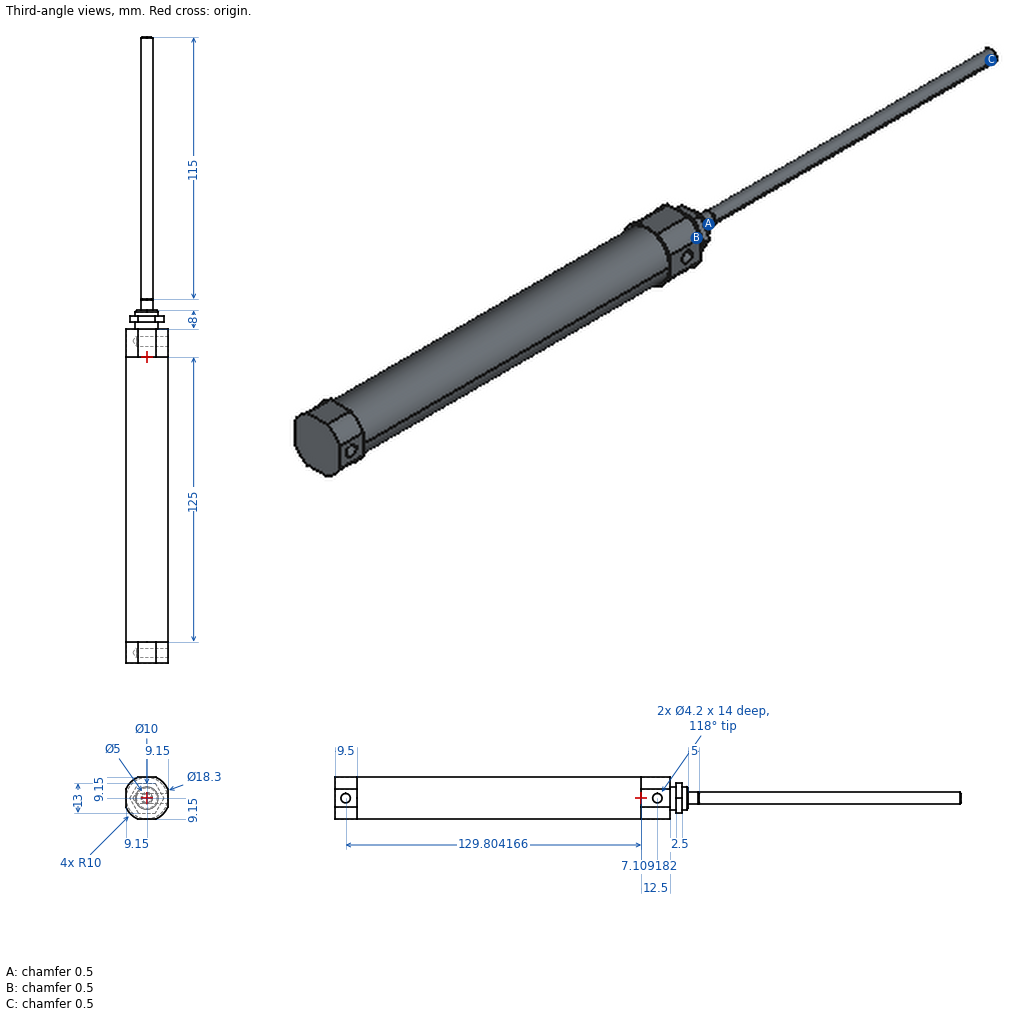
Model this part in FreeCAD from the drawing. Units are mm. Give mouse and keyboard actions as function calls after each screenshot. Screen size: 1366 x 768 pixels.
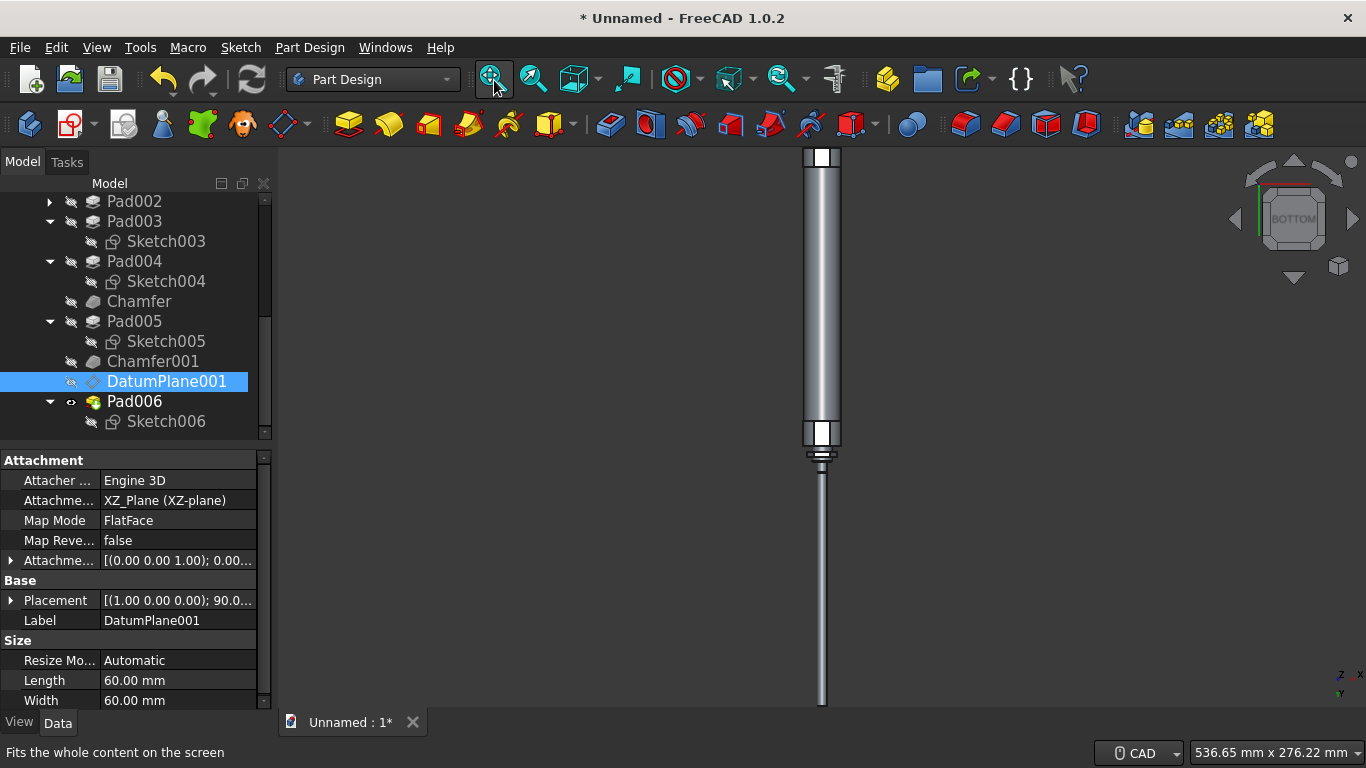
key(4)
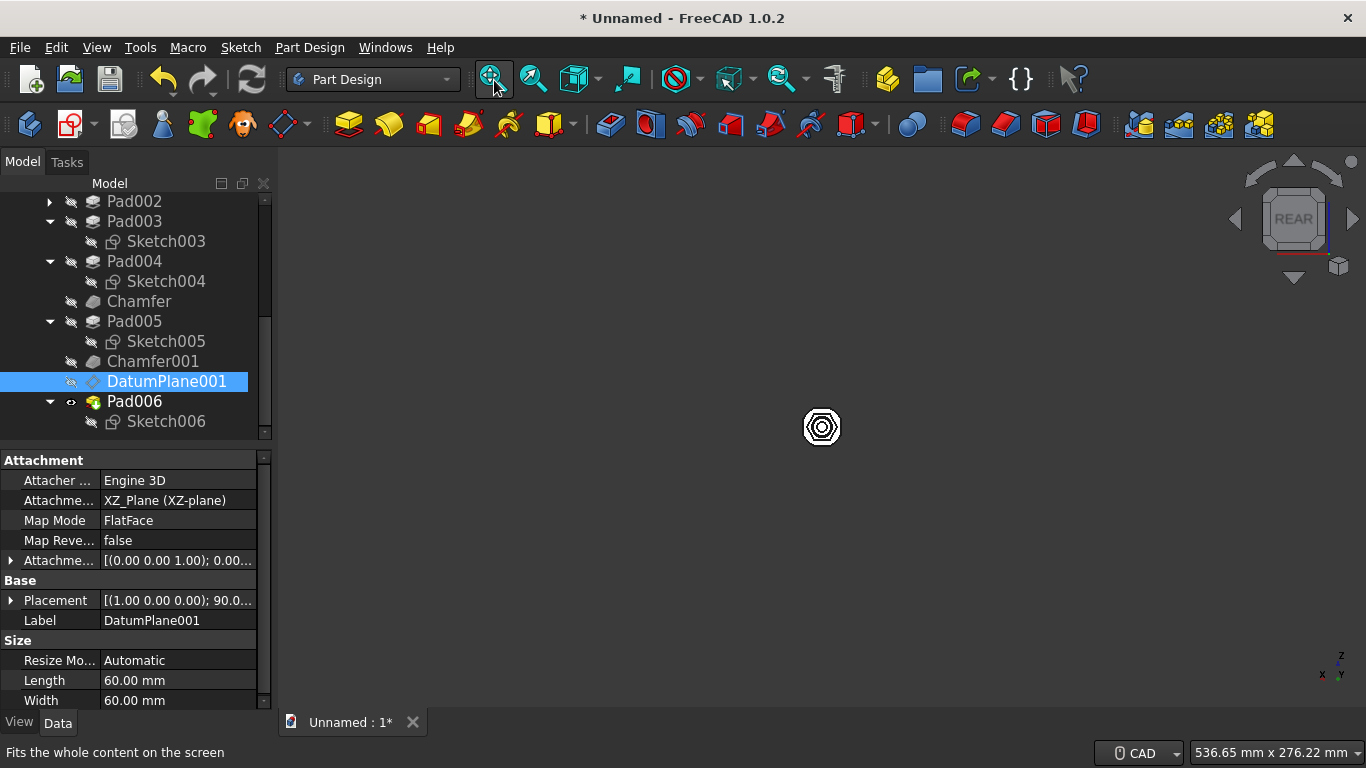
key(v)
key(f)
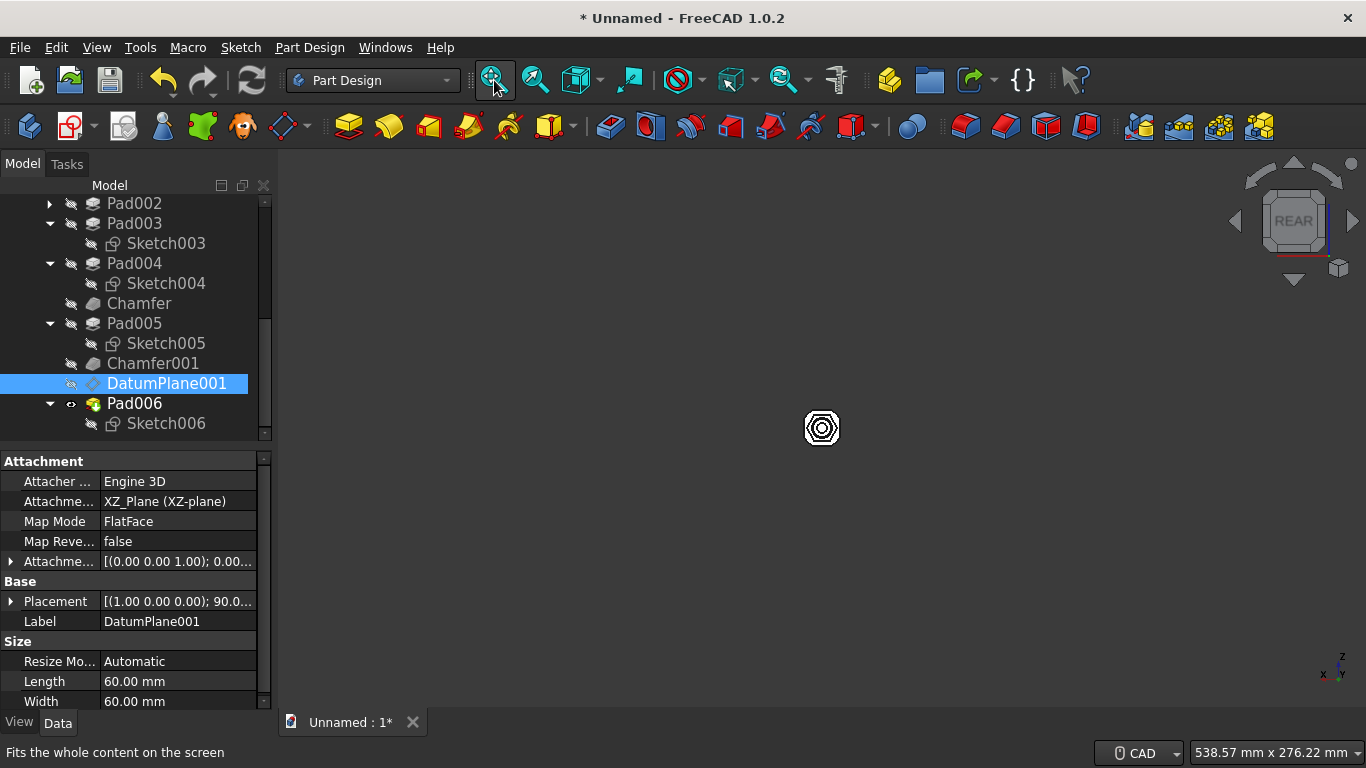
click(827, 427)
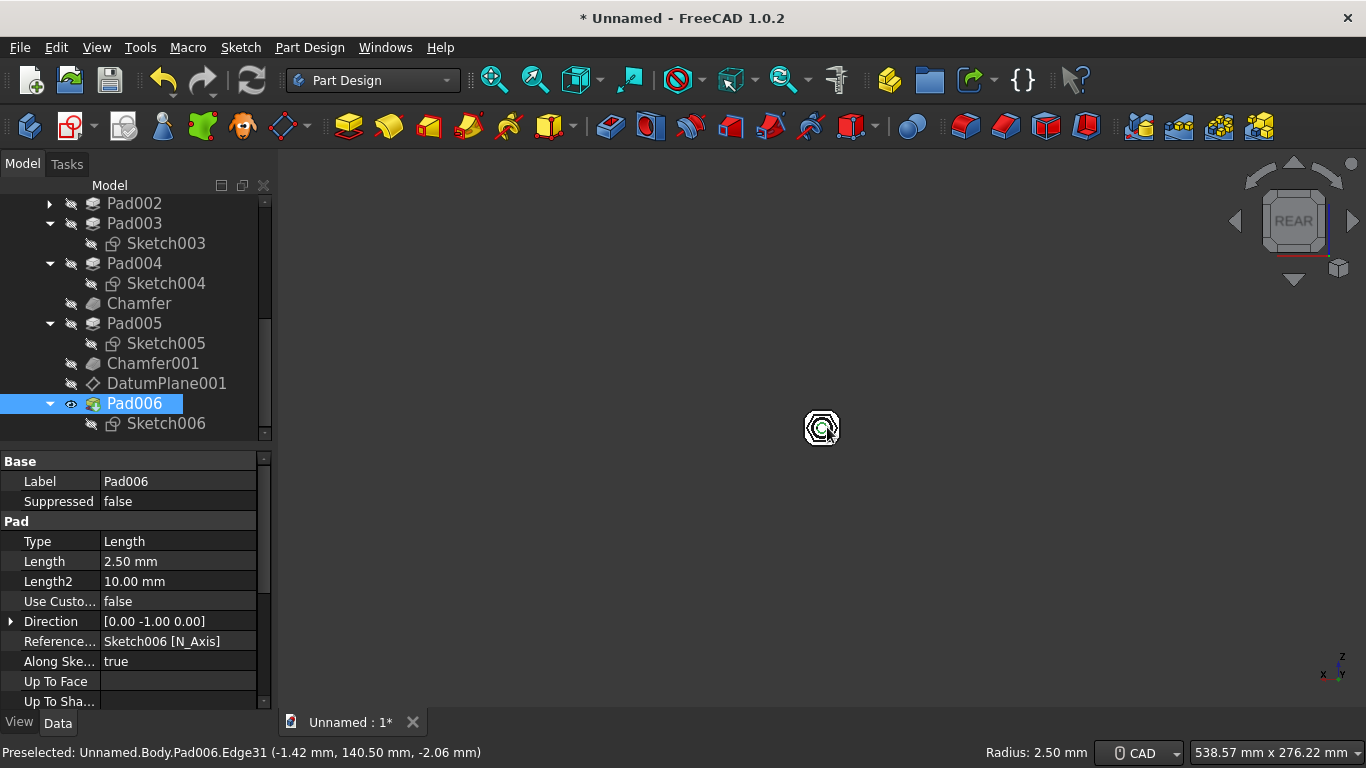
click(1006, 126)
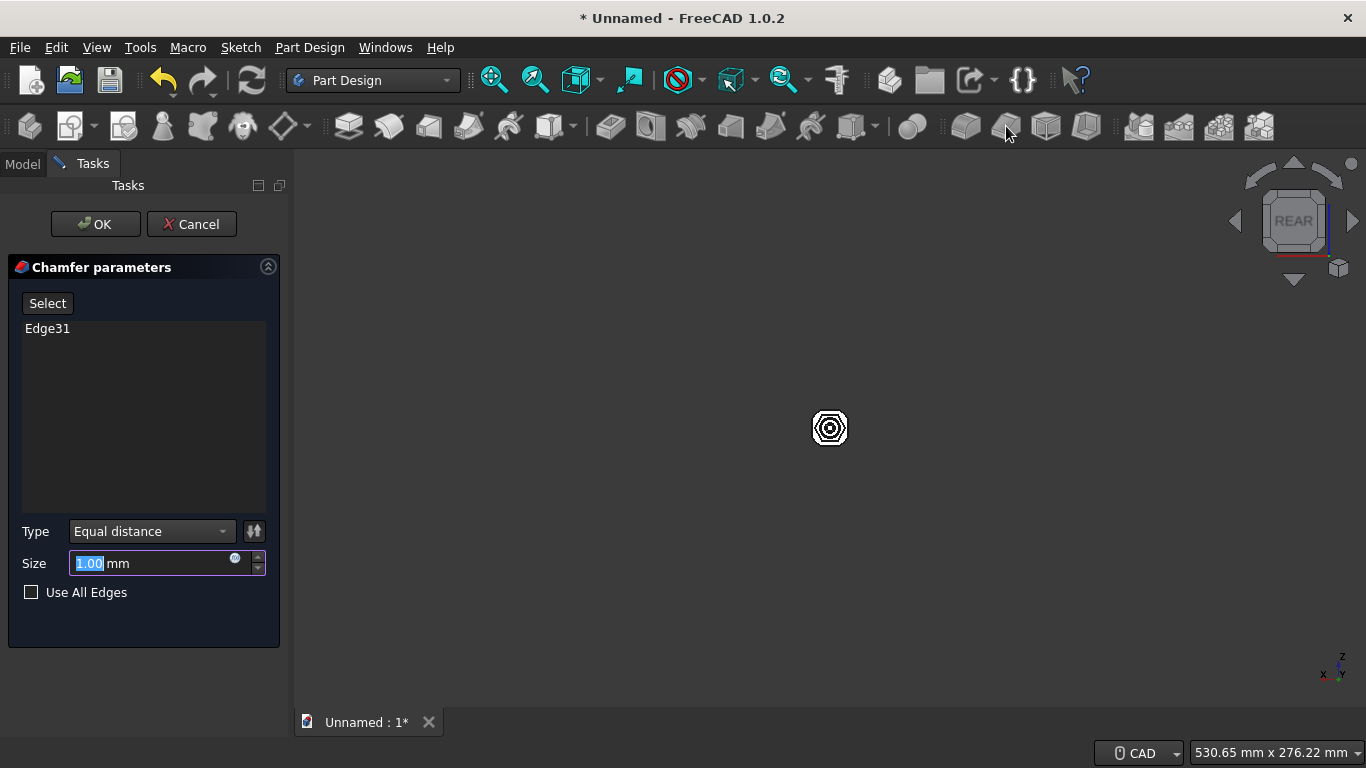
text(0.5)
key(Tab)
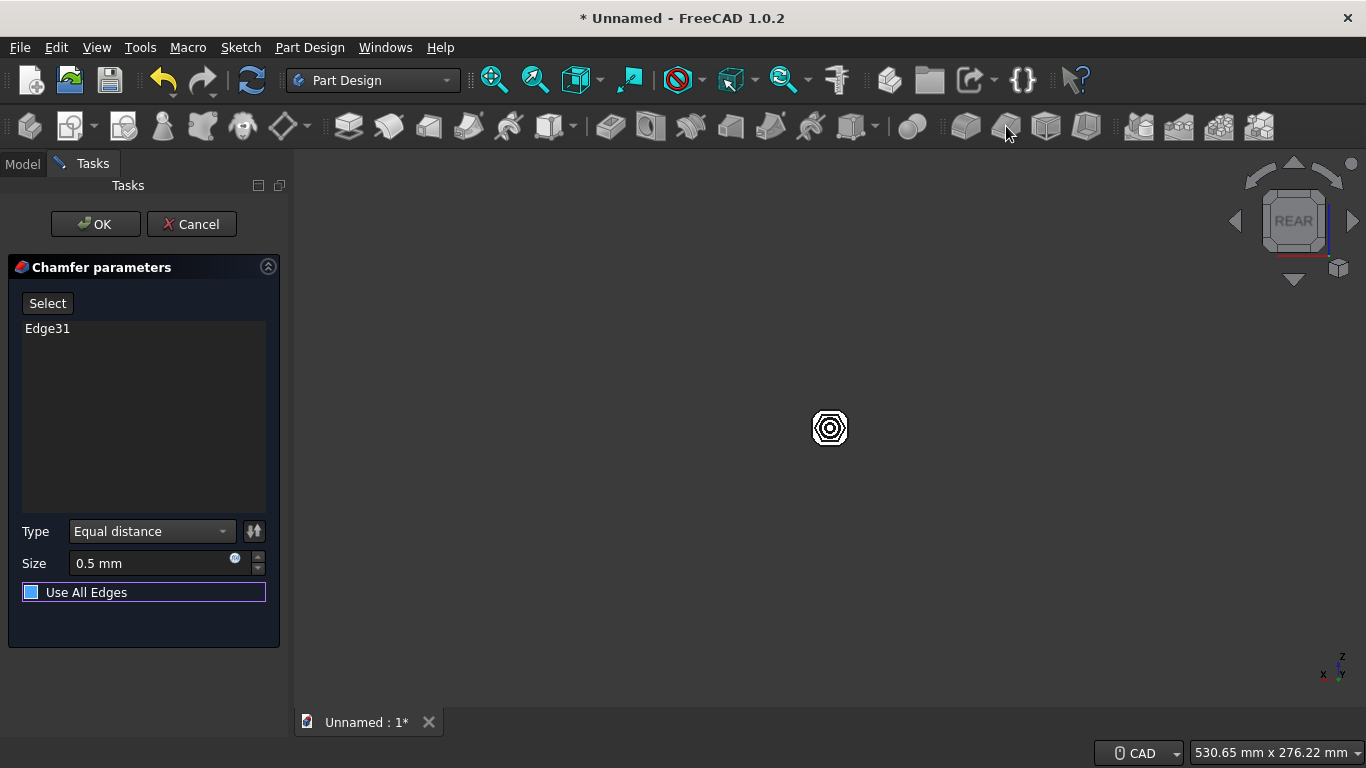
click(96, 224)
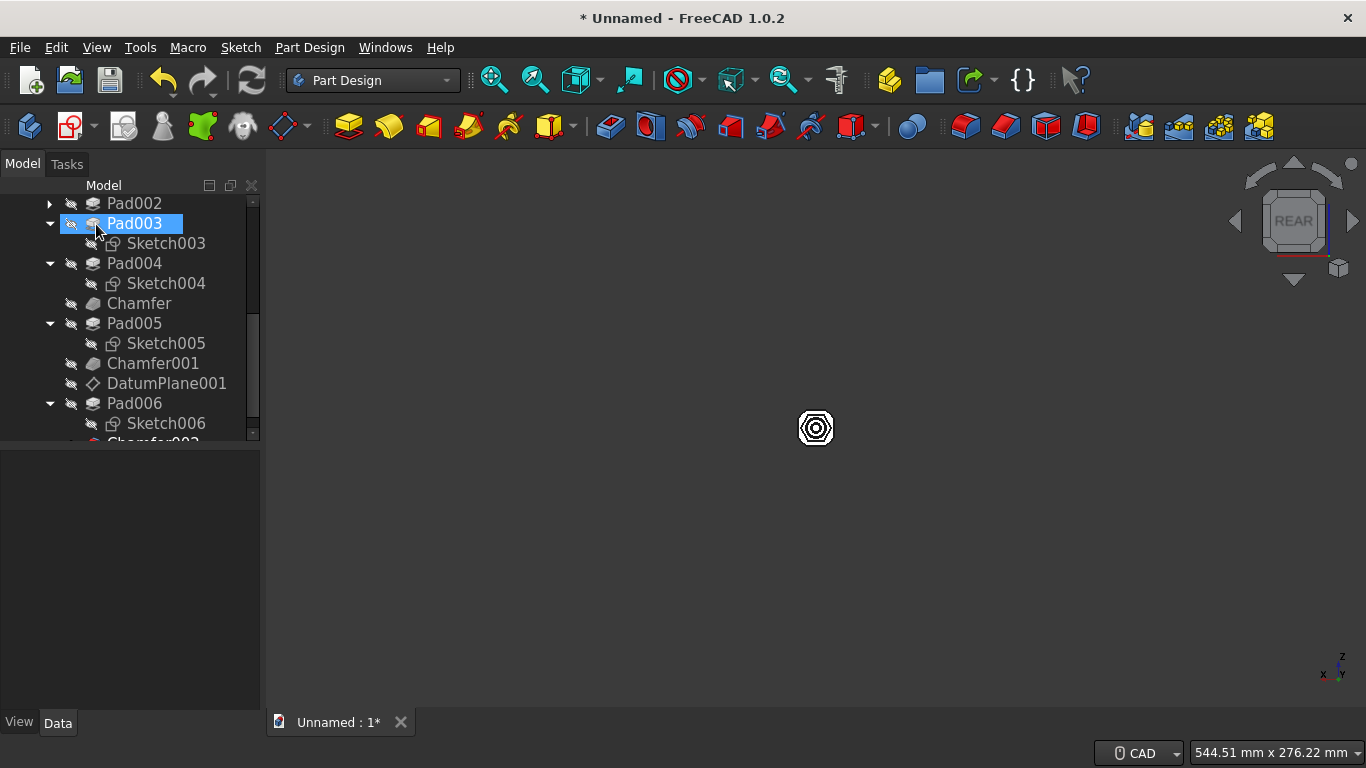
key(v)
key(f)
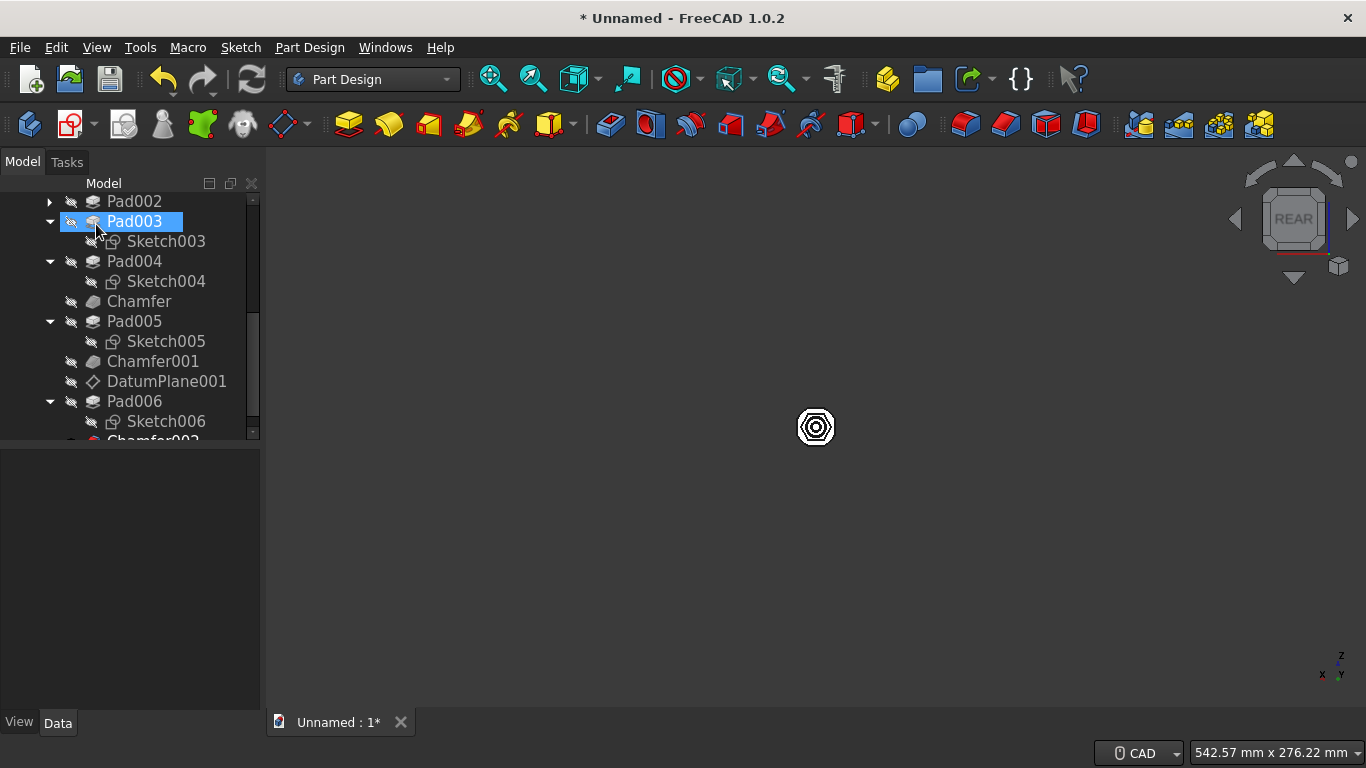
key(0)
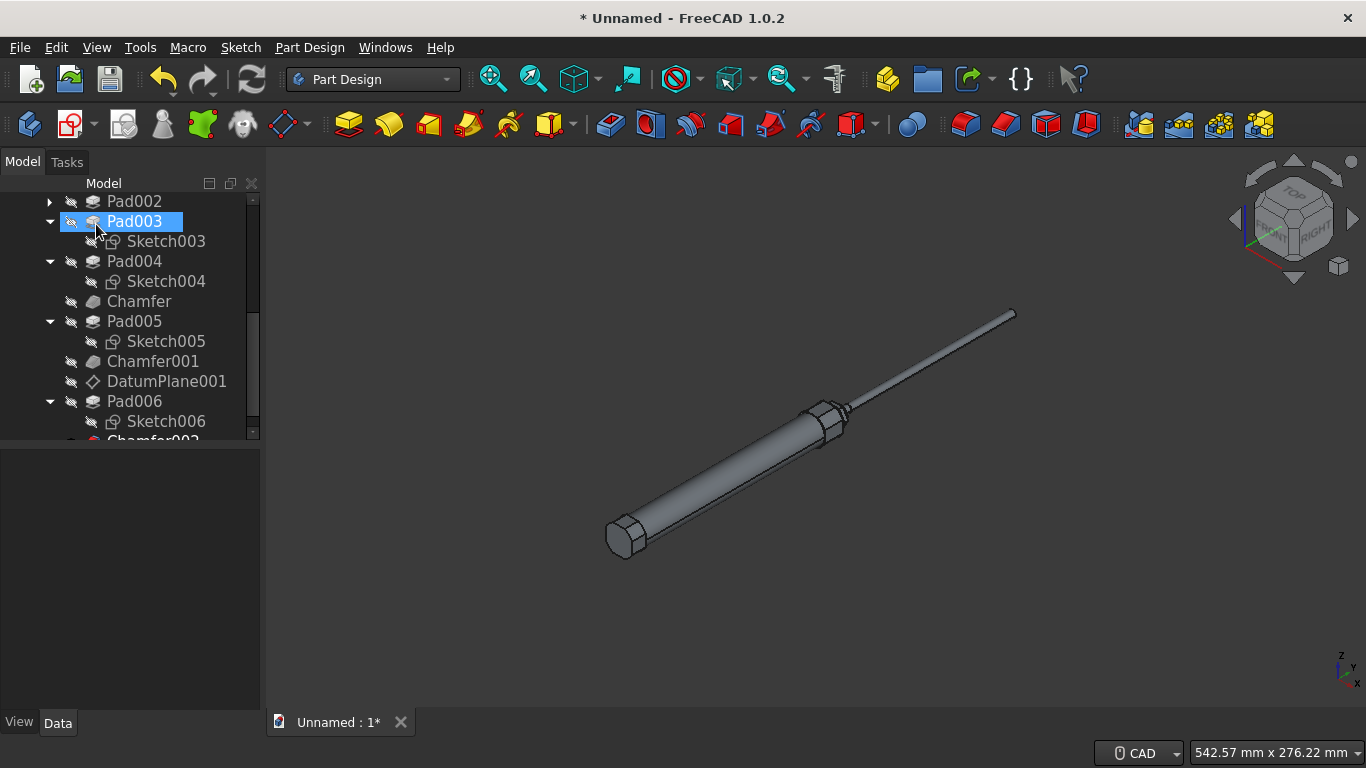
key(3)